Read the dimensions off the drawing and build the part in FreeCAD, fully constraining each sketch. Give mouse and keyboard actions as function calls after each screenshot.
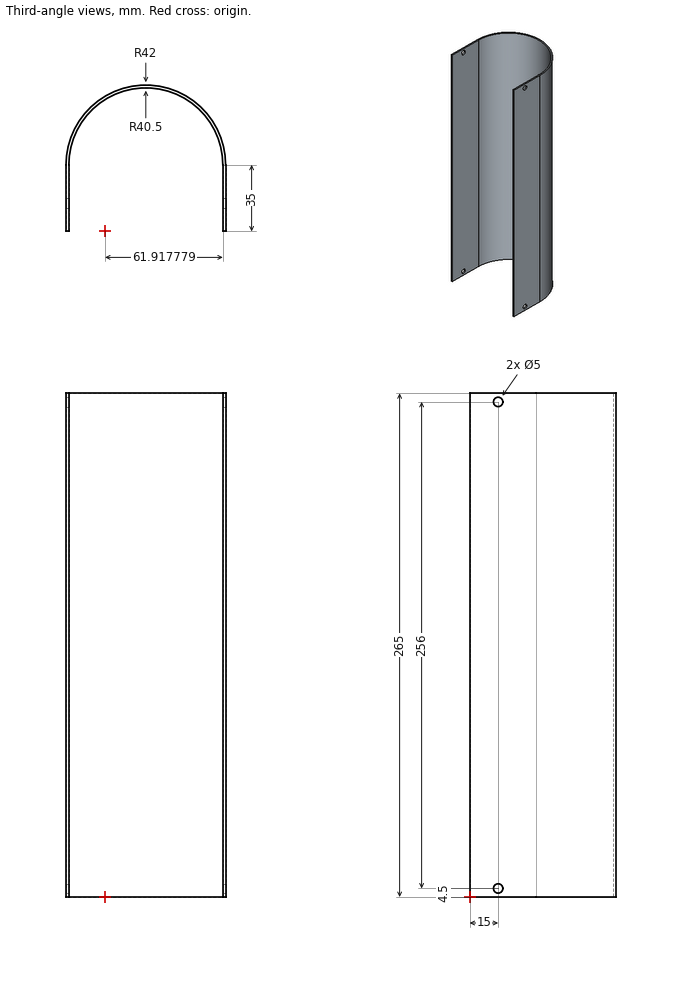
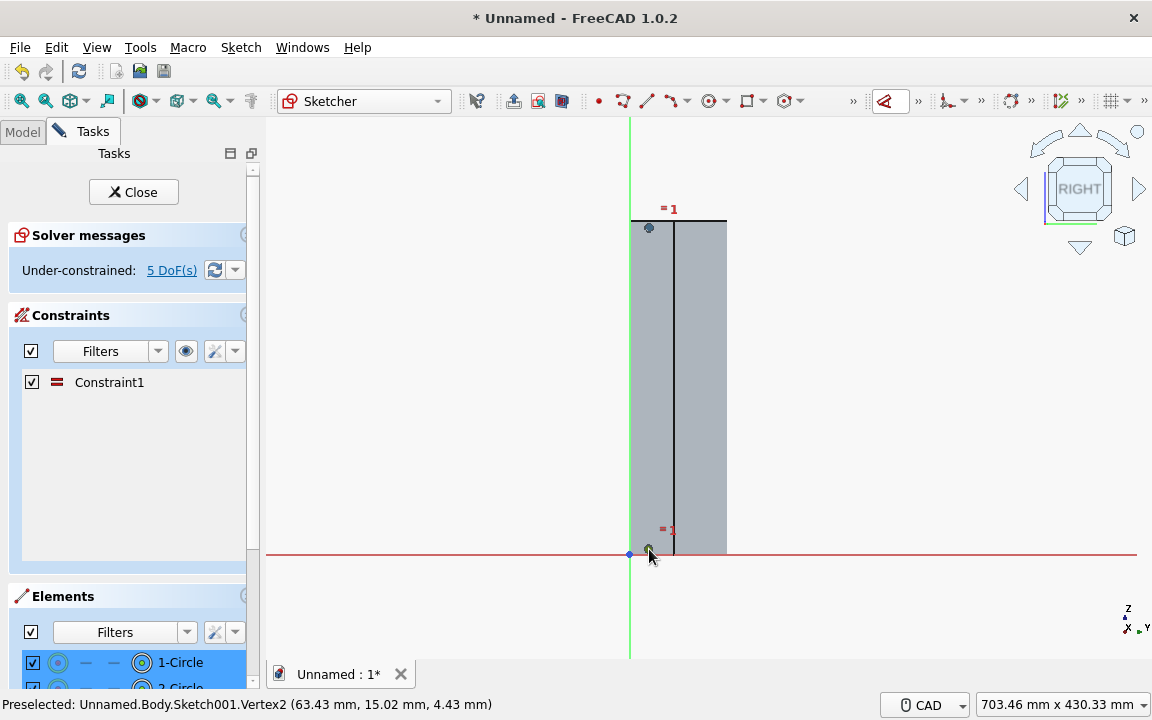
key(v)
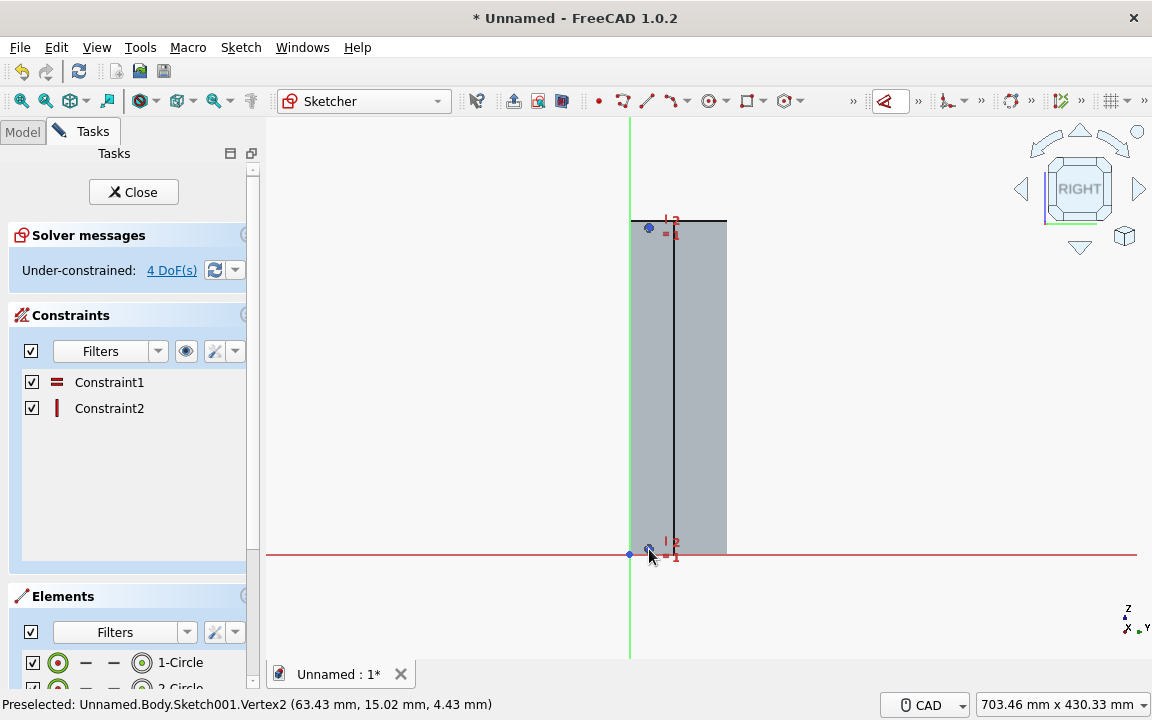
scroll(649, 224, up, 10)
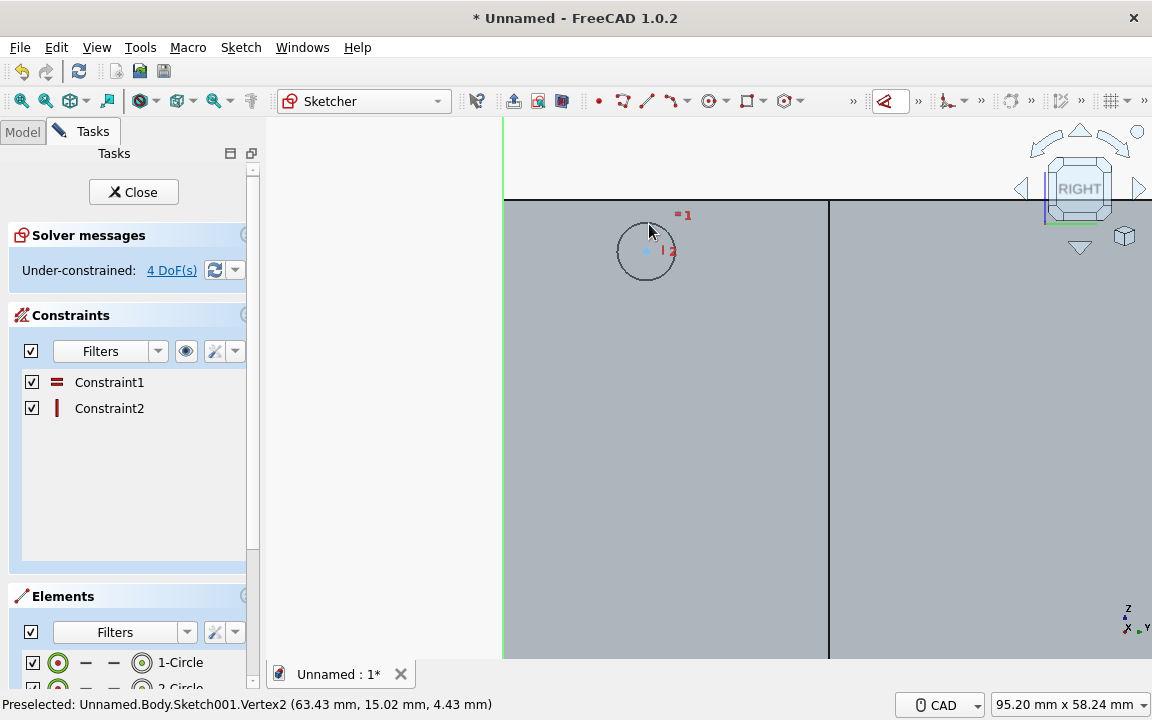
click(647, 223)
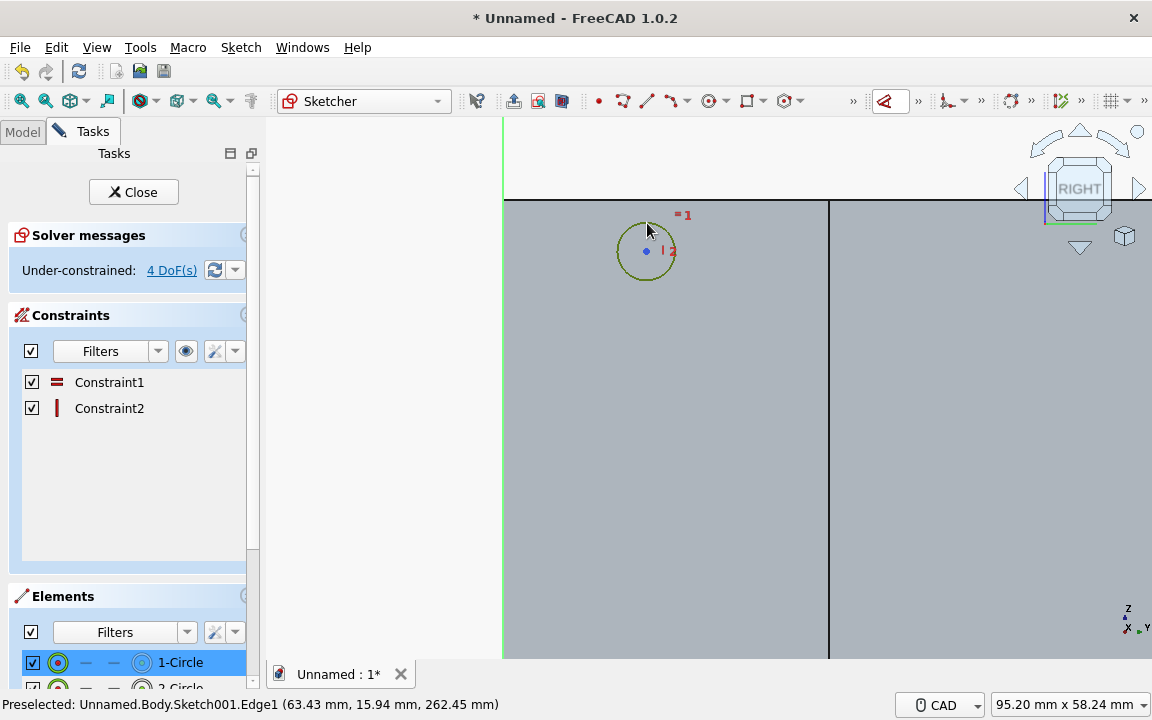
key(k)
key(o)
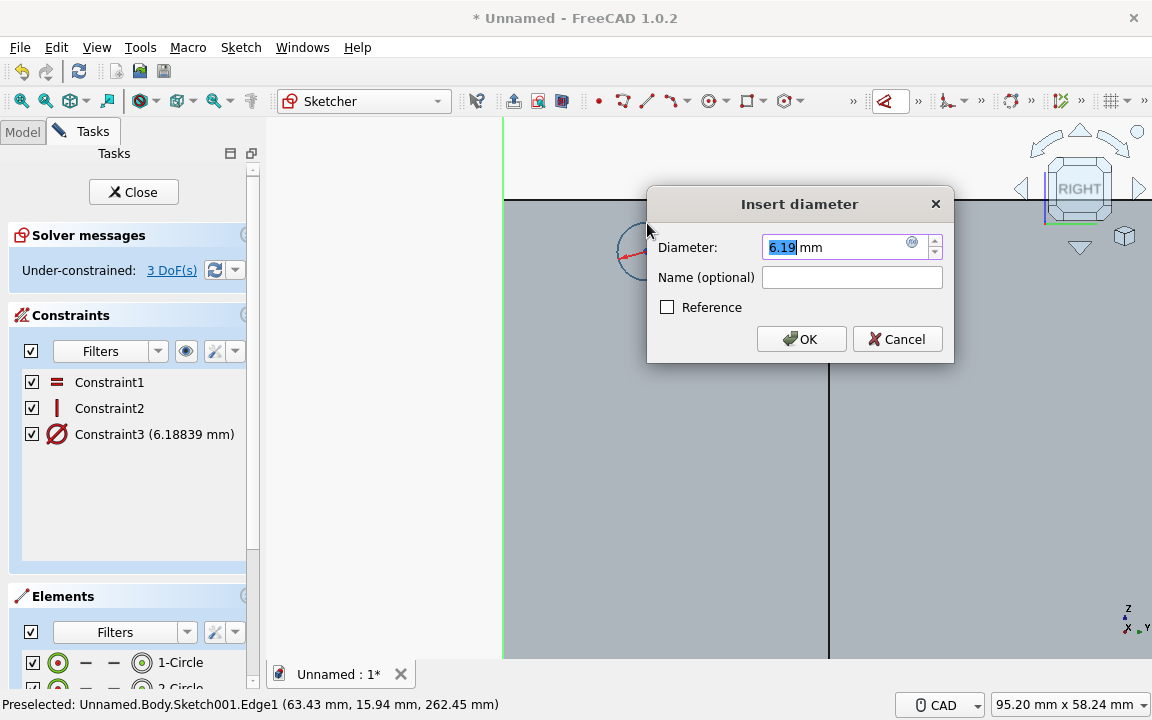
text(5)
key(Return)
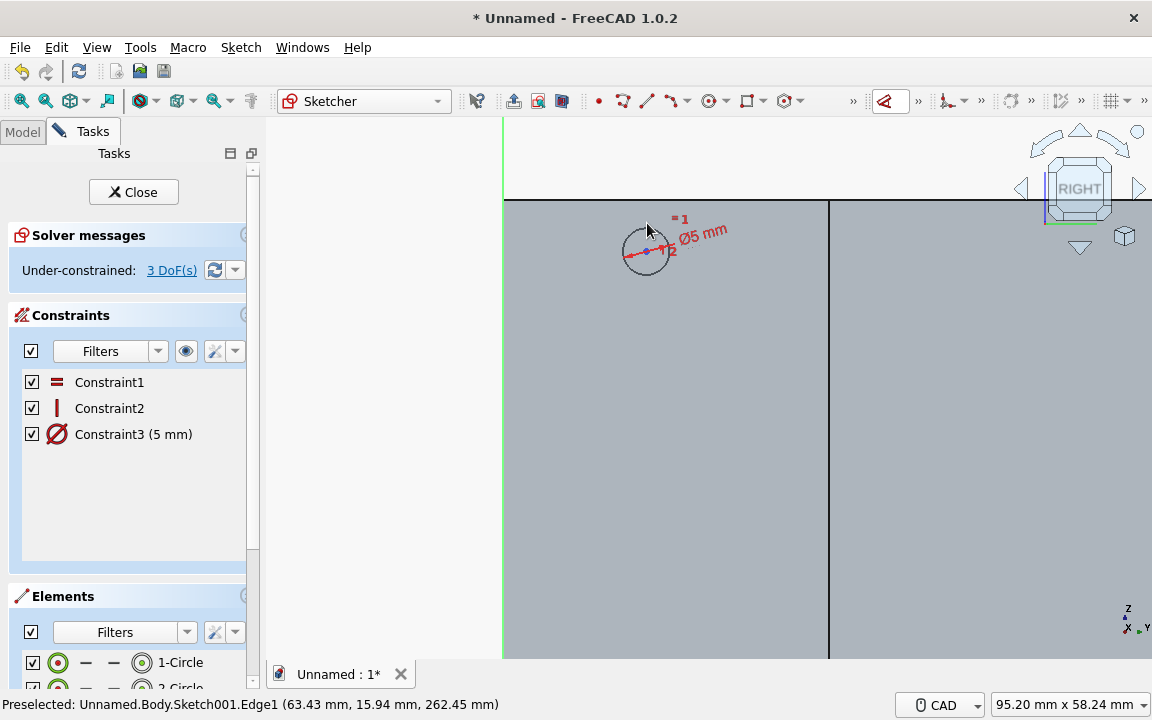
scroll(649, 223, down, 10)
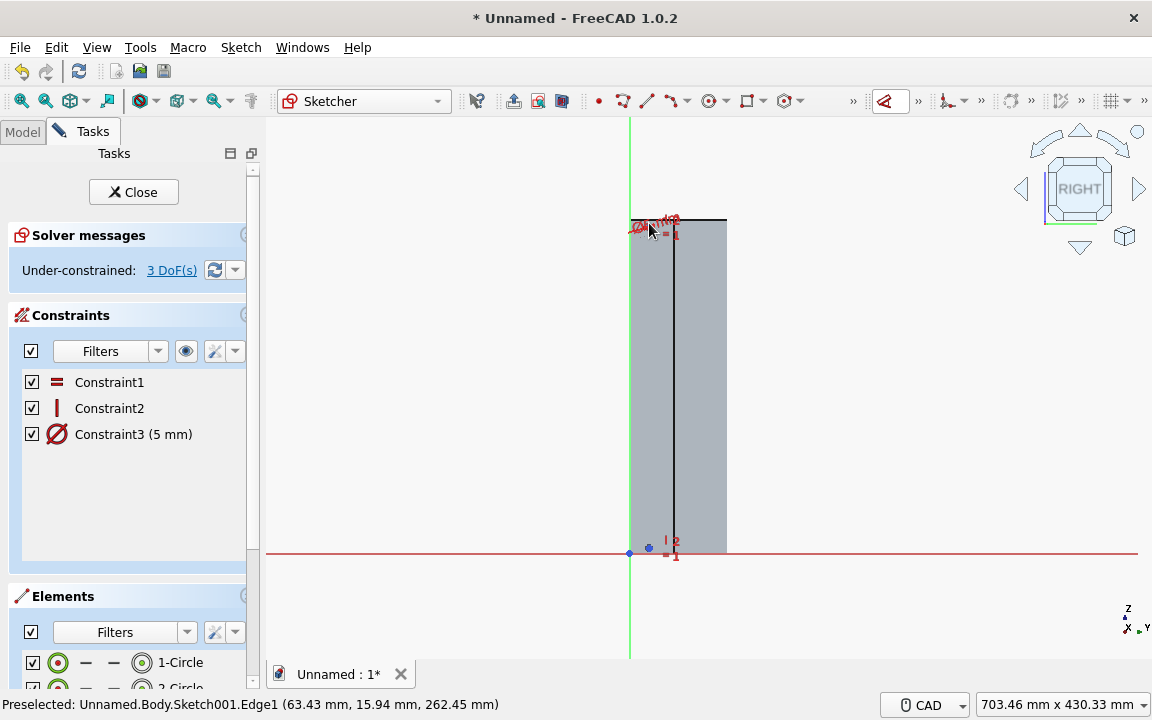
scroll(649, 227, up, 4)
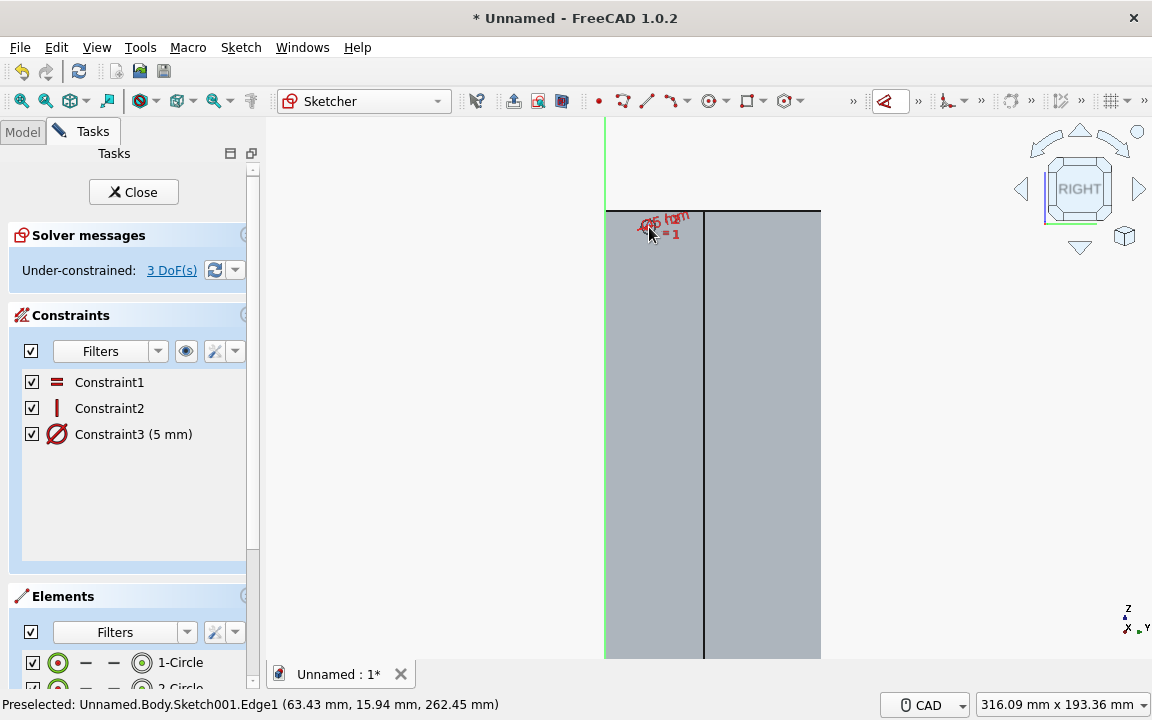
click(648, 227)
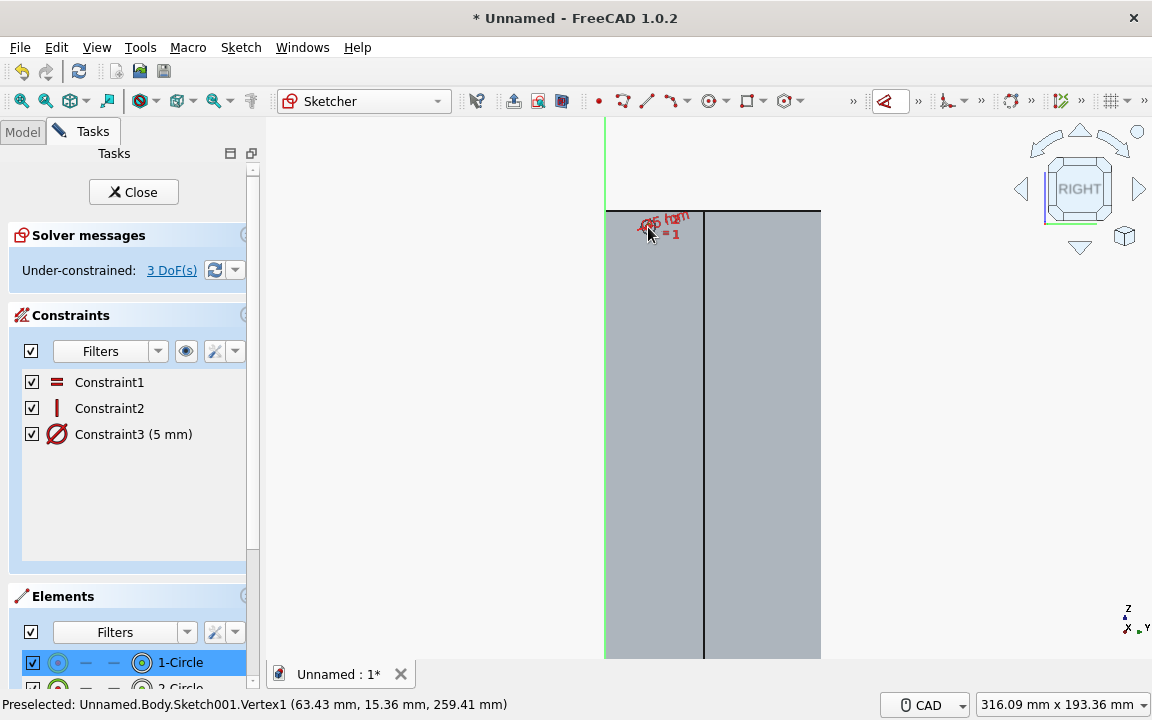
key(l)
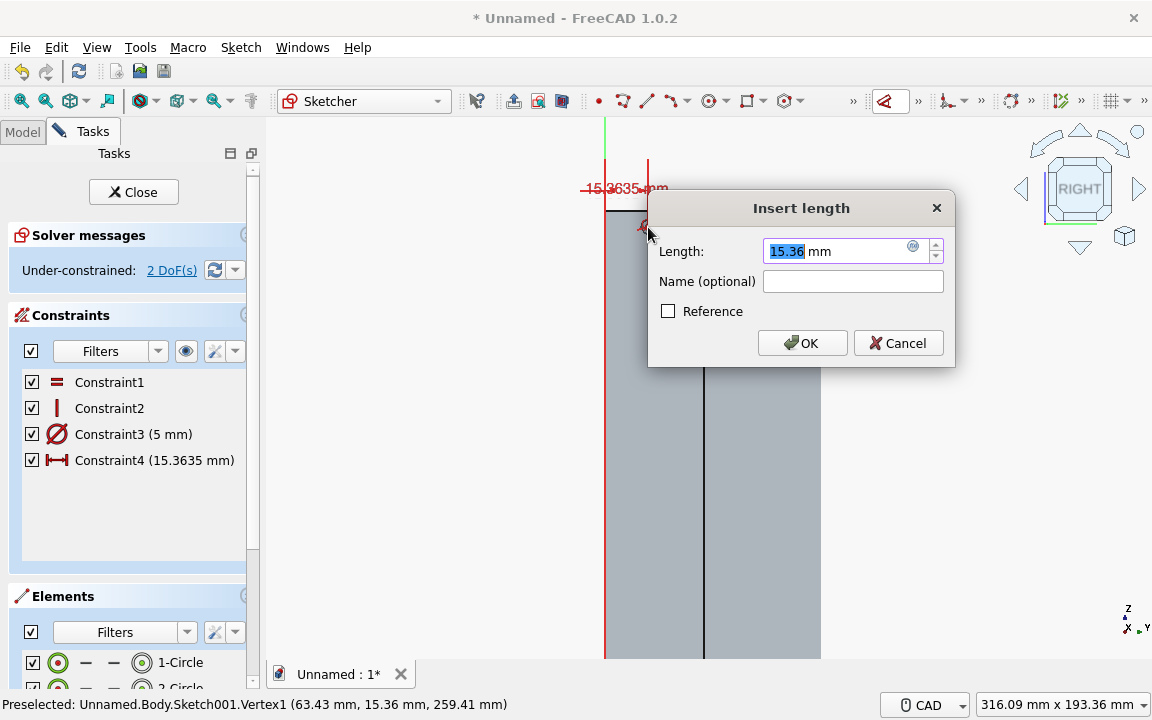
text(15)
key(Return)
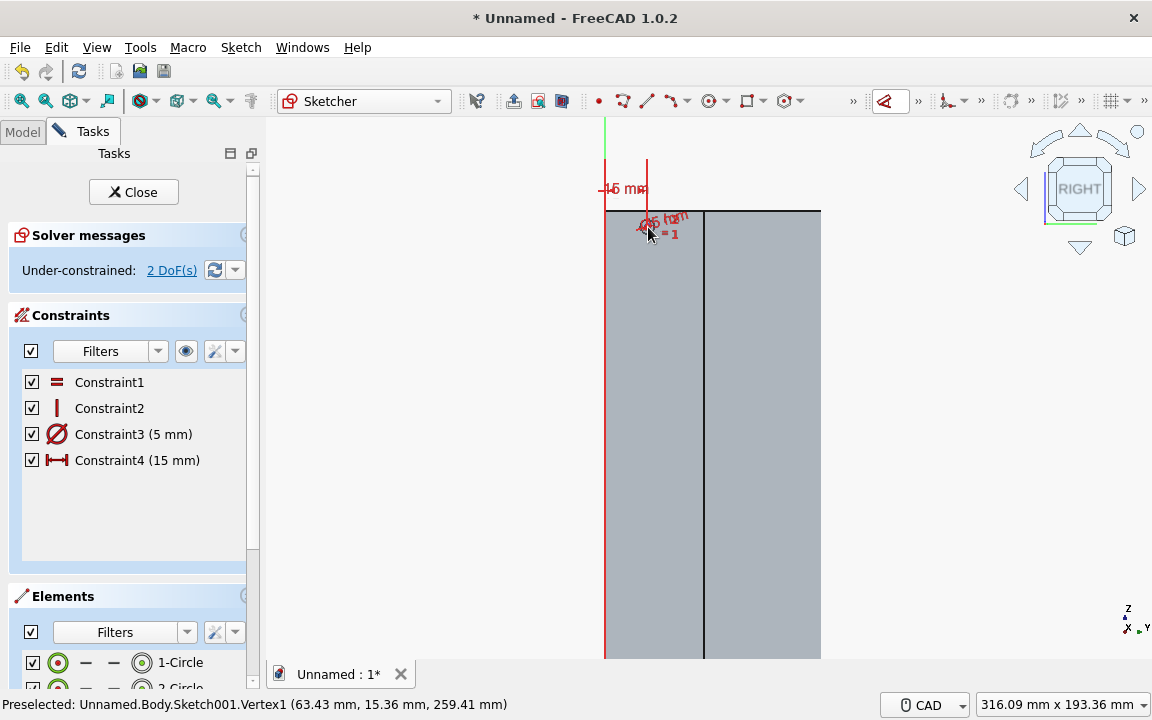
scroll(649, 227, down, 4)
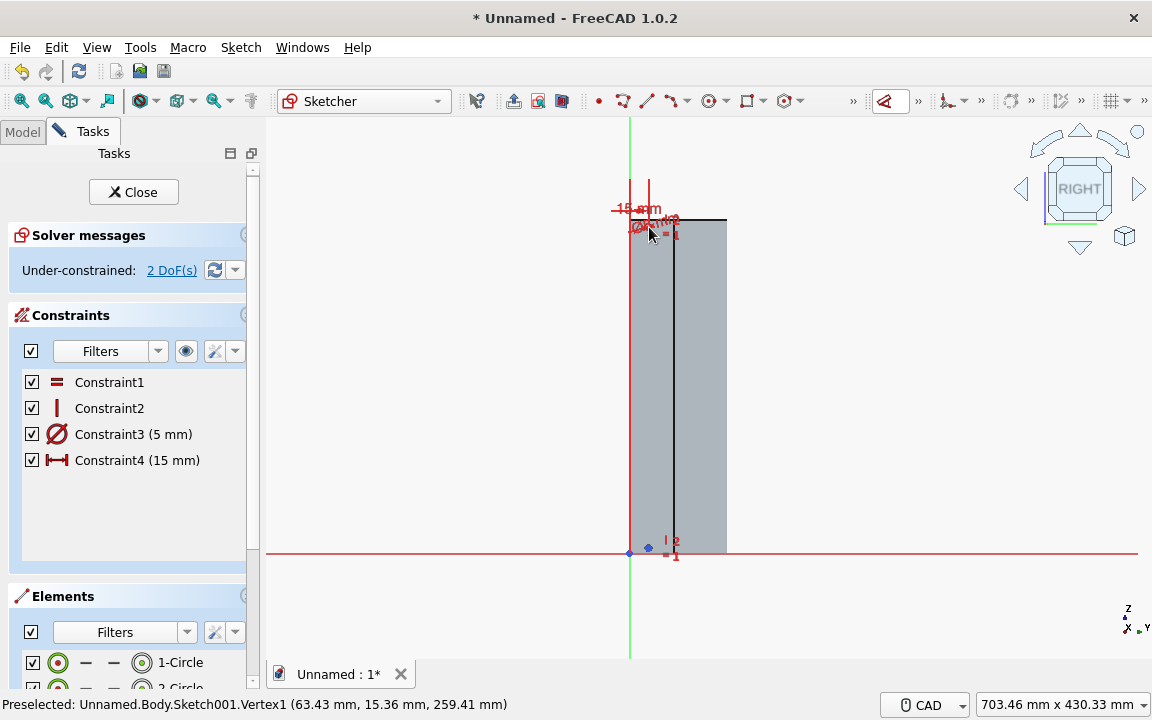
scroll(649, 548, up, 10)